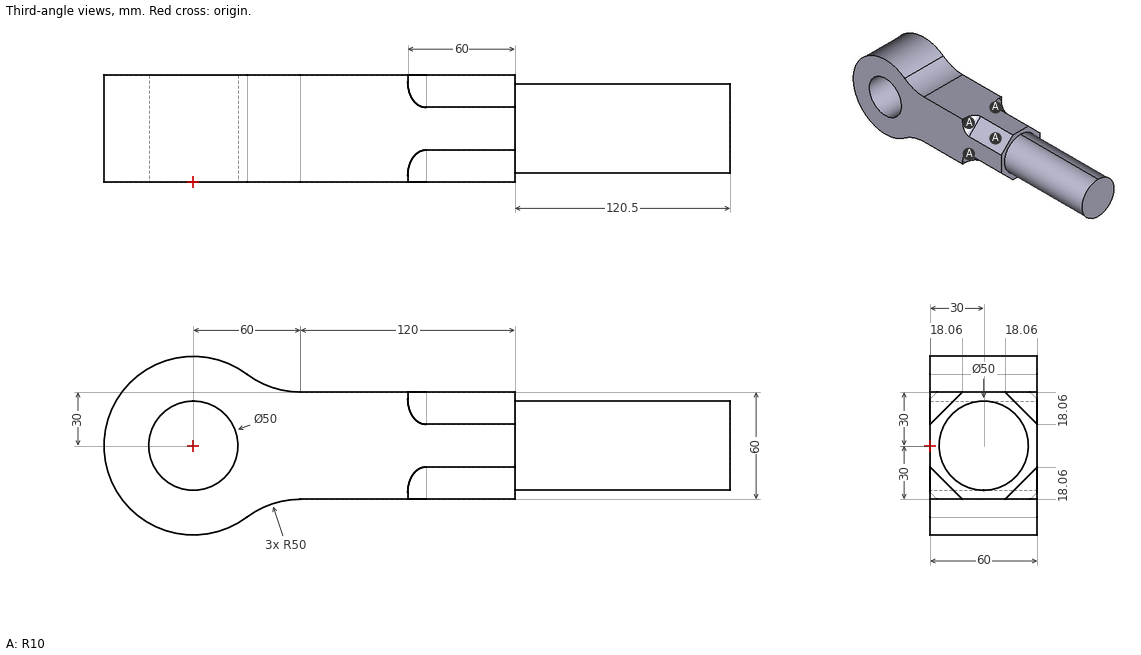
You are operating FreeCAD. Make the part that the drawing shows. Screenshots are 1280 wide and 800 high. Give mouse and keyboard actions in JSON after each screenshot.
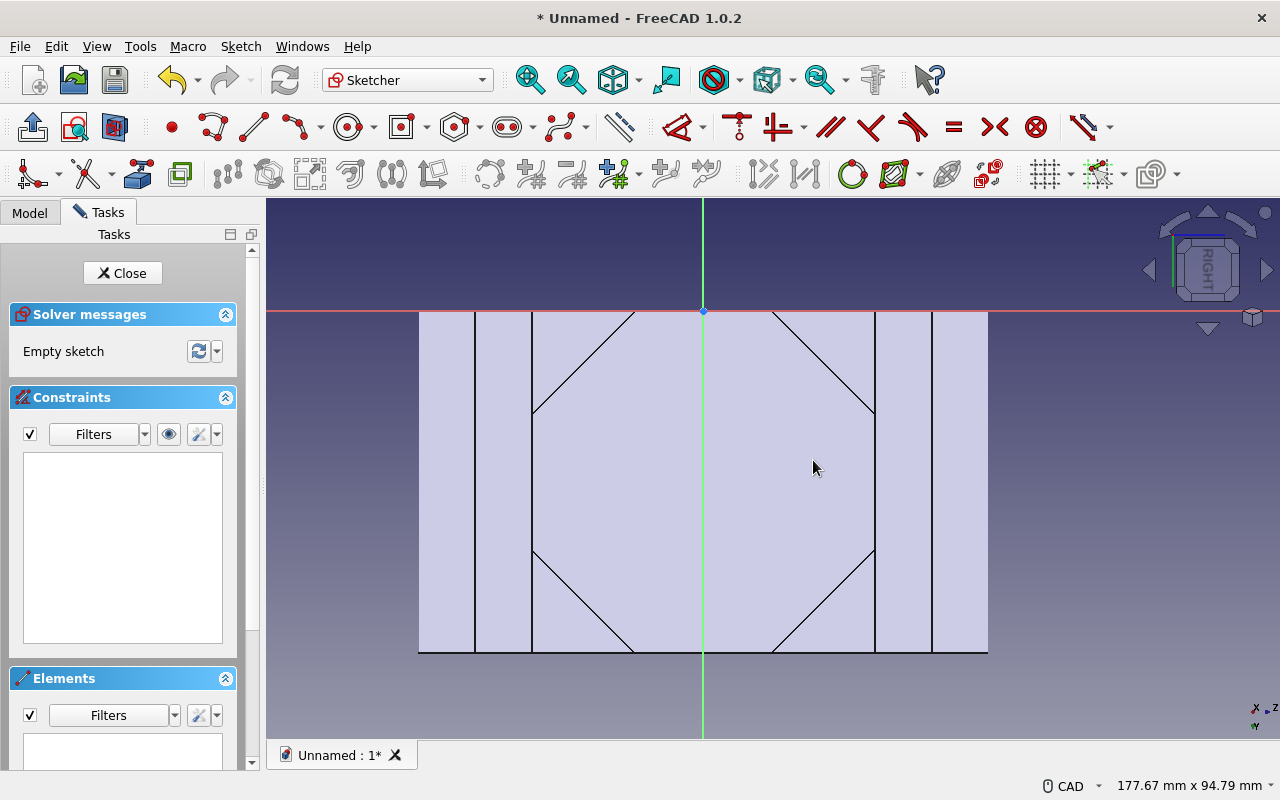
{"action": "key", "text": "g c"}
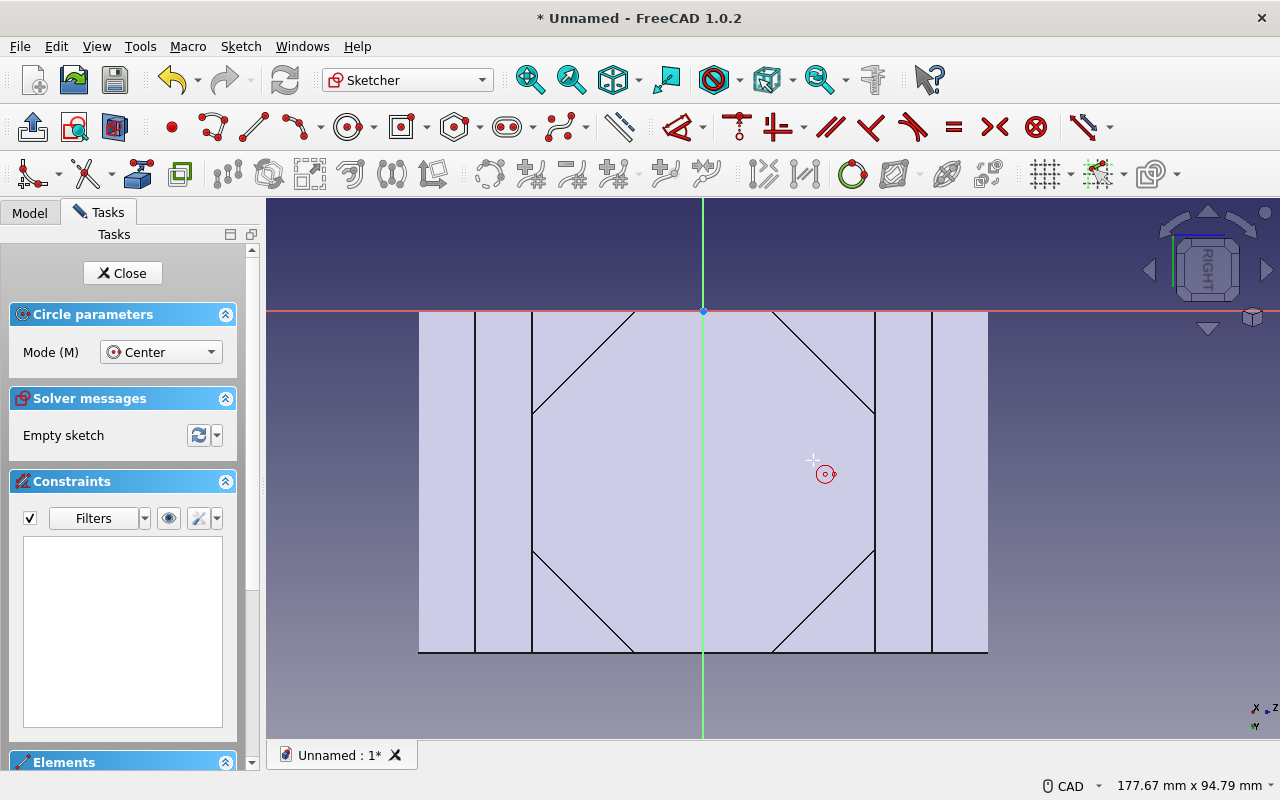
{"action": "left_click", "coordinate": [703, 482]}
{"action": "mouse_move", "coordinate": [804, 381]}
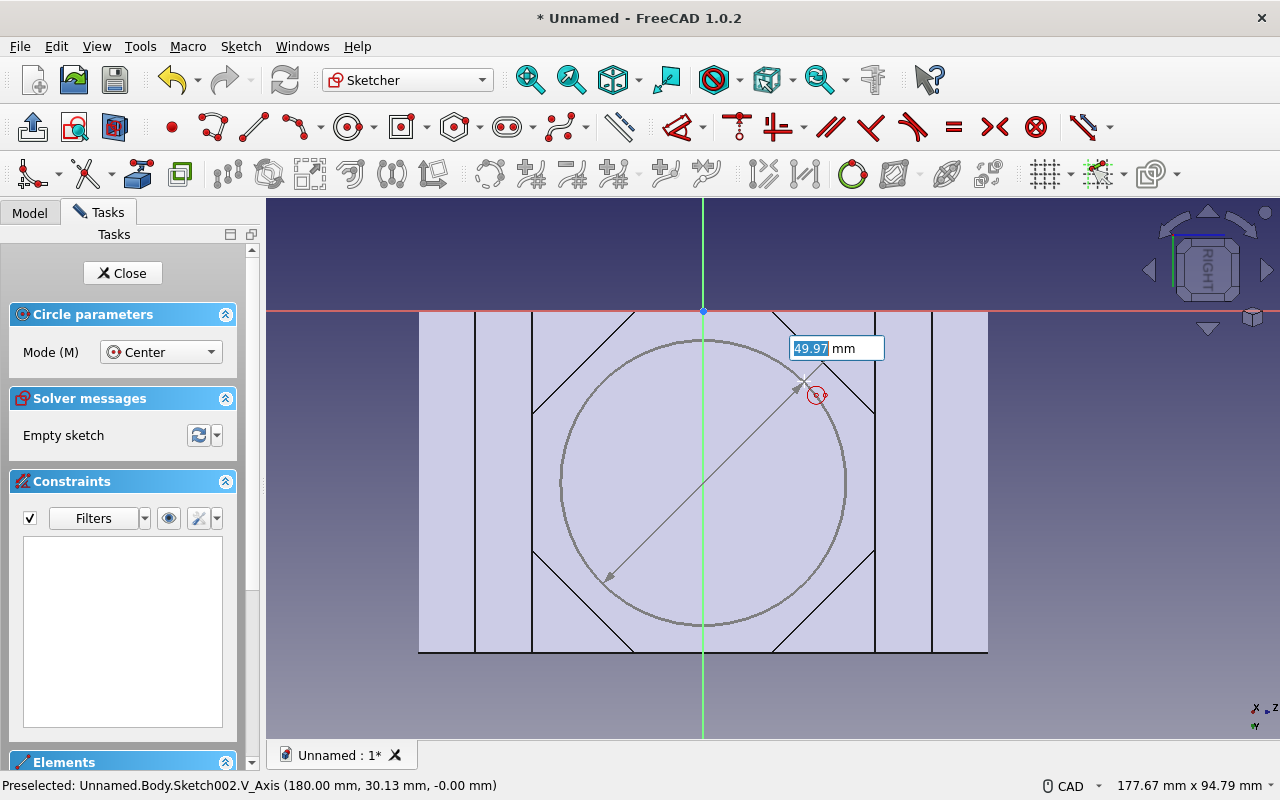
{"action": "type", "text": "50"}
{"action": "key", "text": "Return"}
{"action": "key", "text": "Escape"}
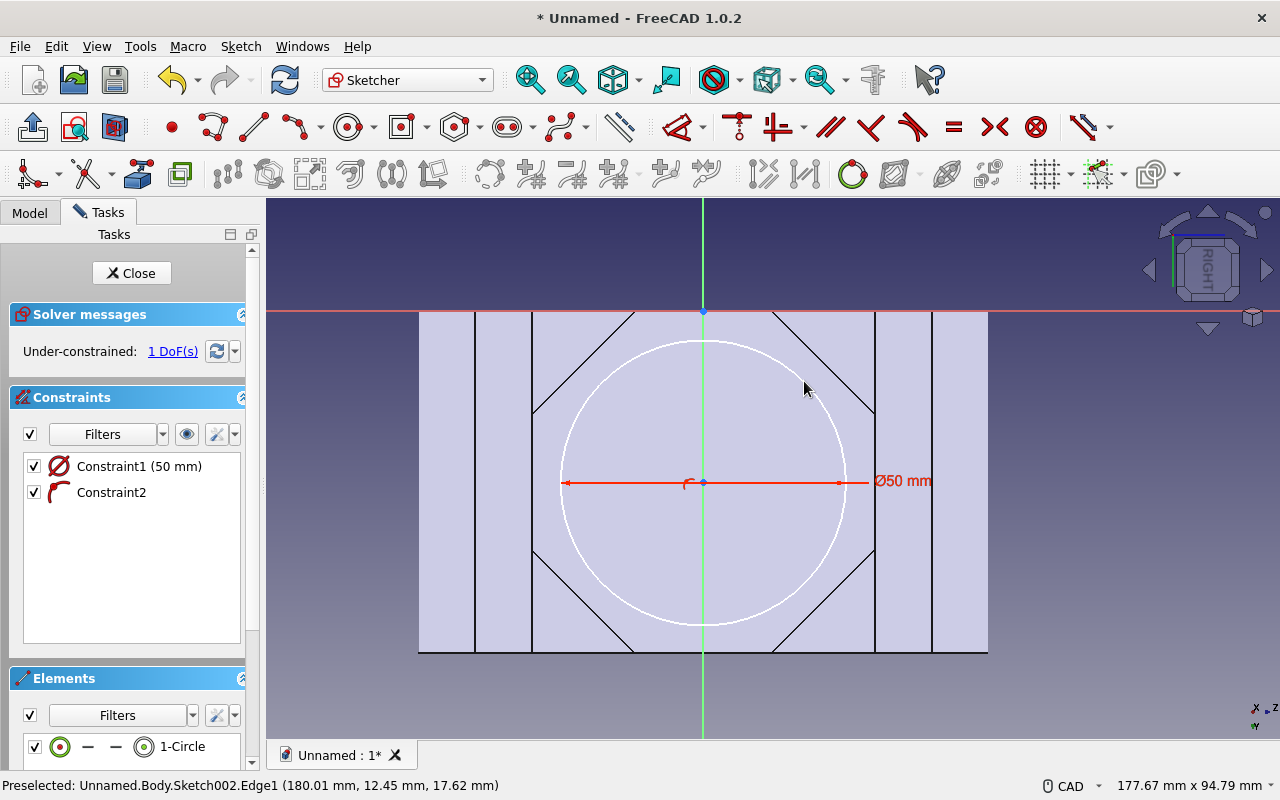
{"action": "key", "text": "d"}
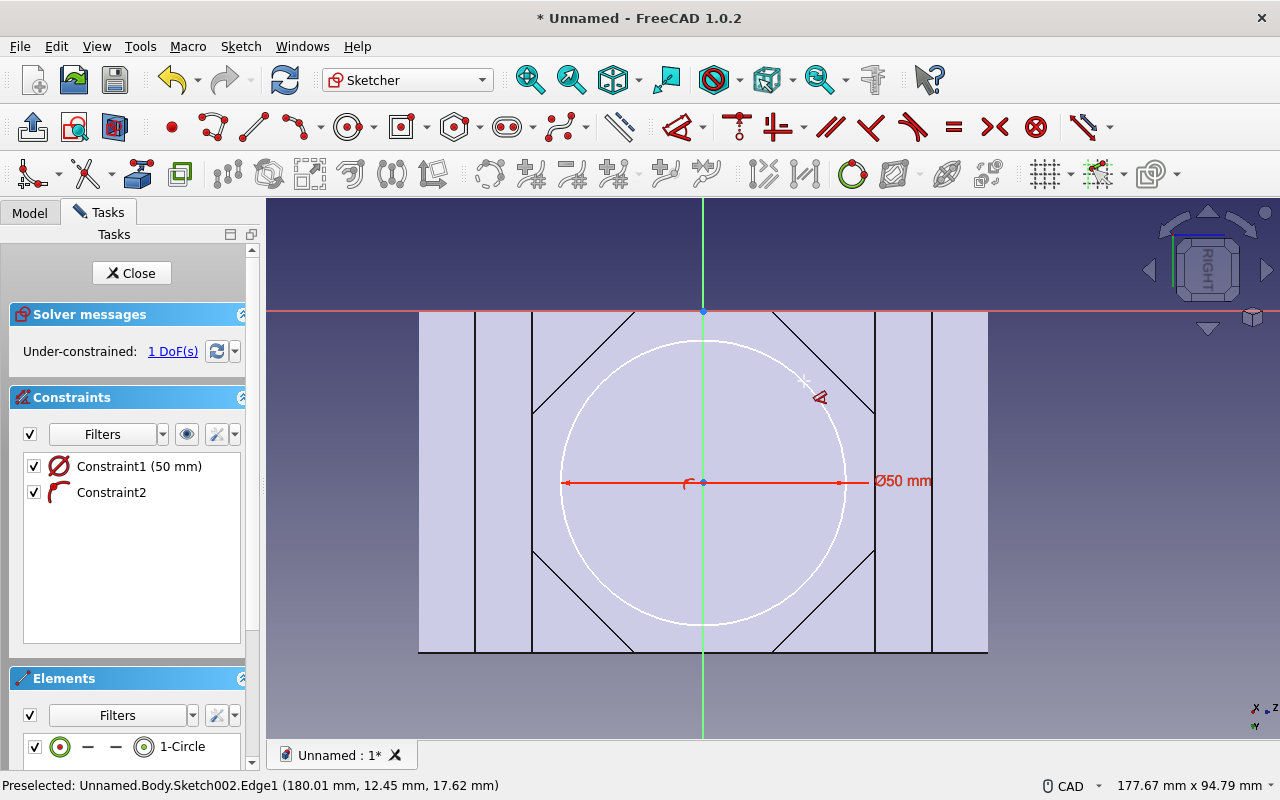
{"action": "left_click", "coordinate": [703, 483]}
{"action": "left_click", "coordinate": [737, 397]}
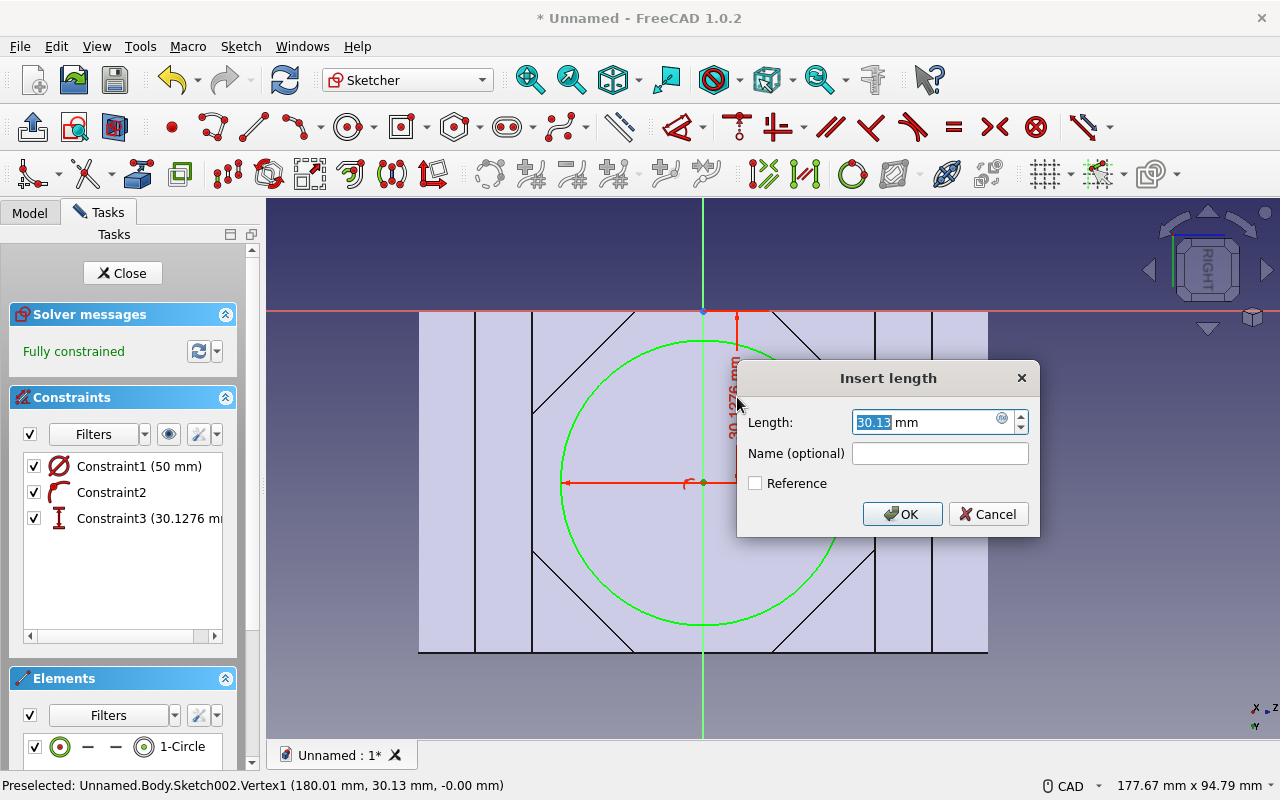
{"action": "type", "text": "30"}
{"action": "key", "text": "Return"}
{"action": "key", "text": "Escape"}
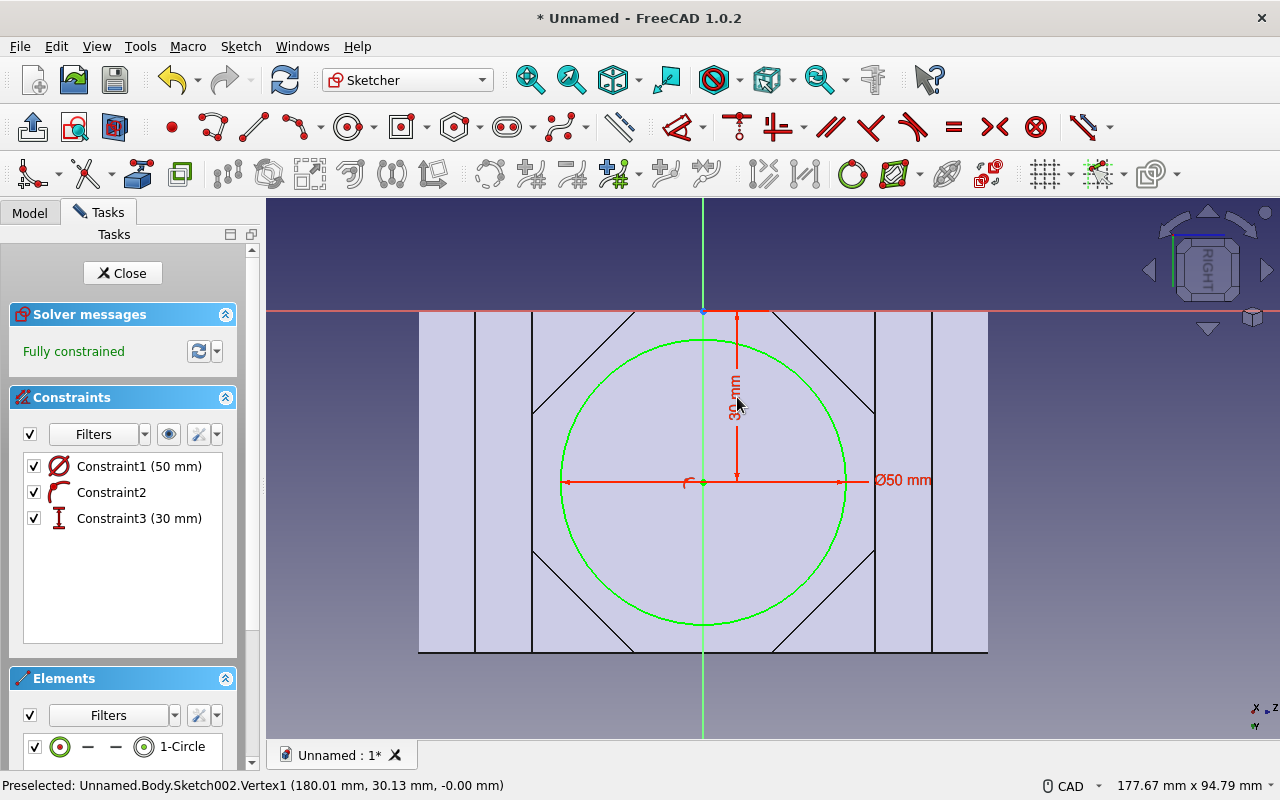
{"action": "left_click", "coordinate": [123, 273]}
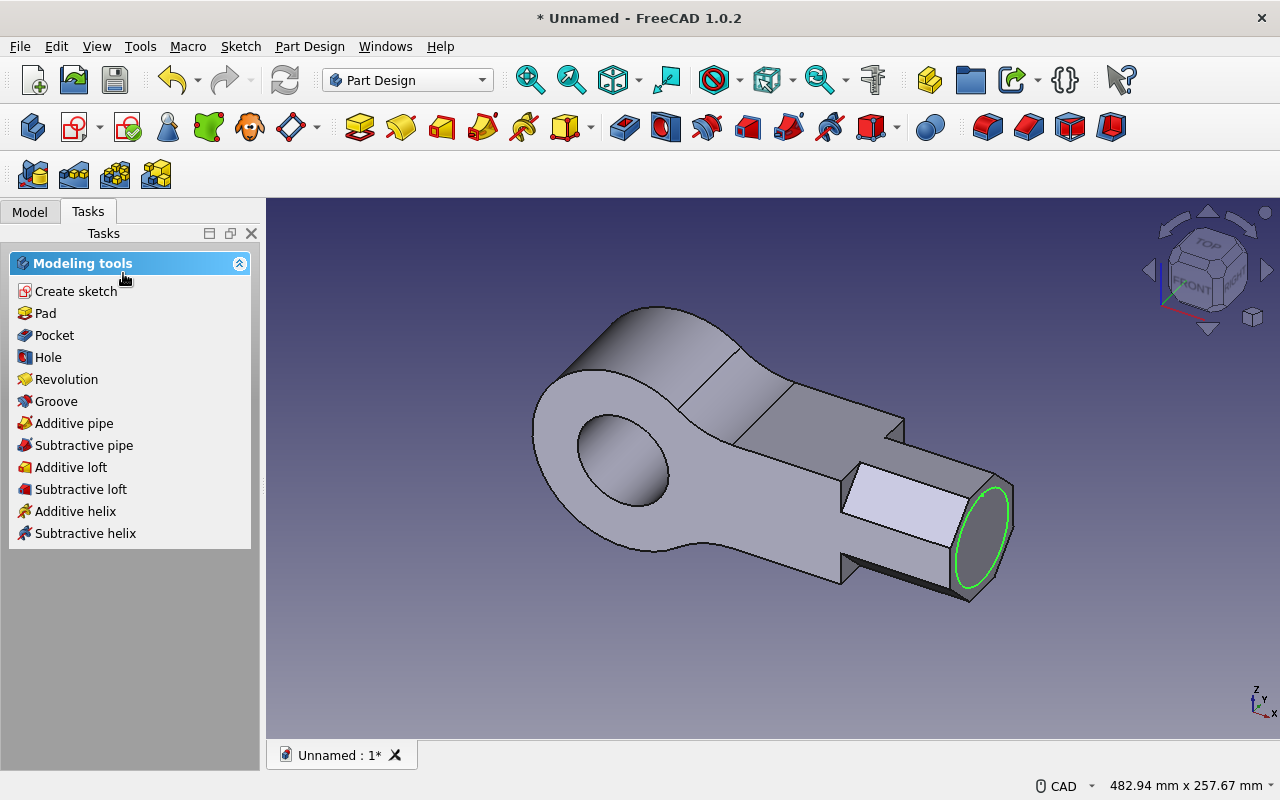
{"action": "left_click", "coordinate": [360, 128]}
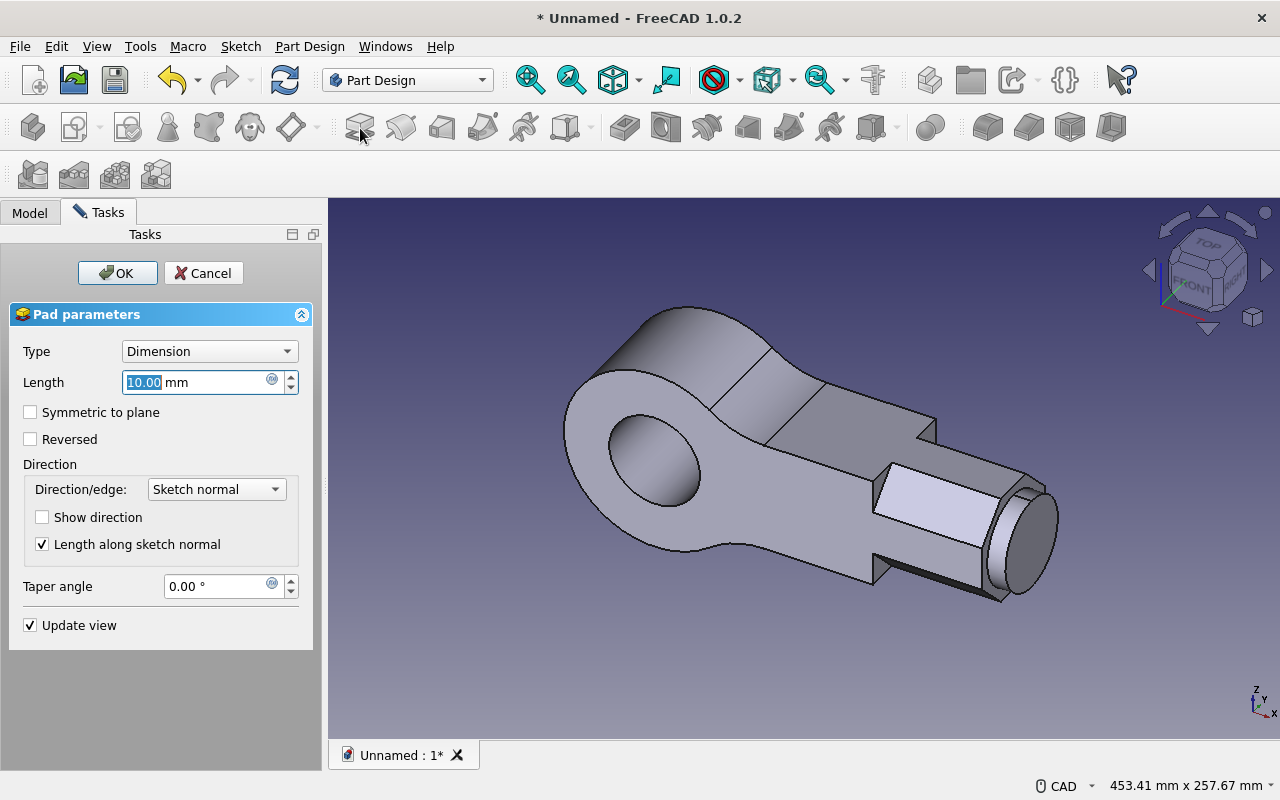
{"action": "type", "text": "120.5"}
{"action": "key", "text": "Tab"}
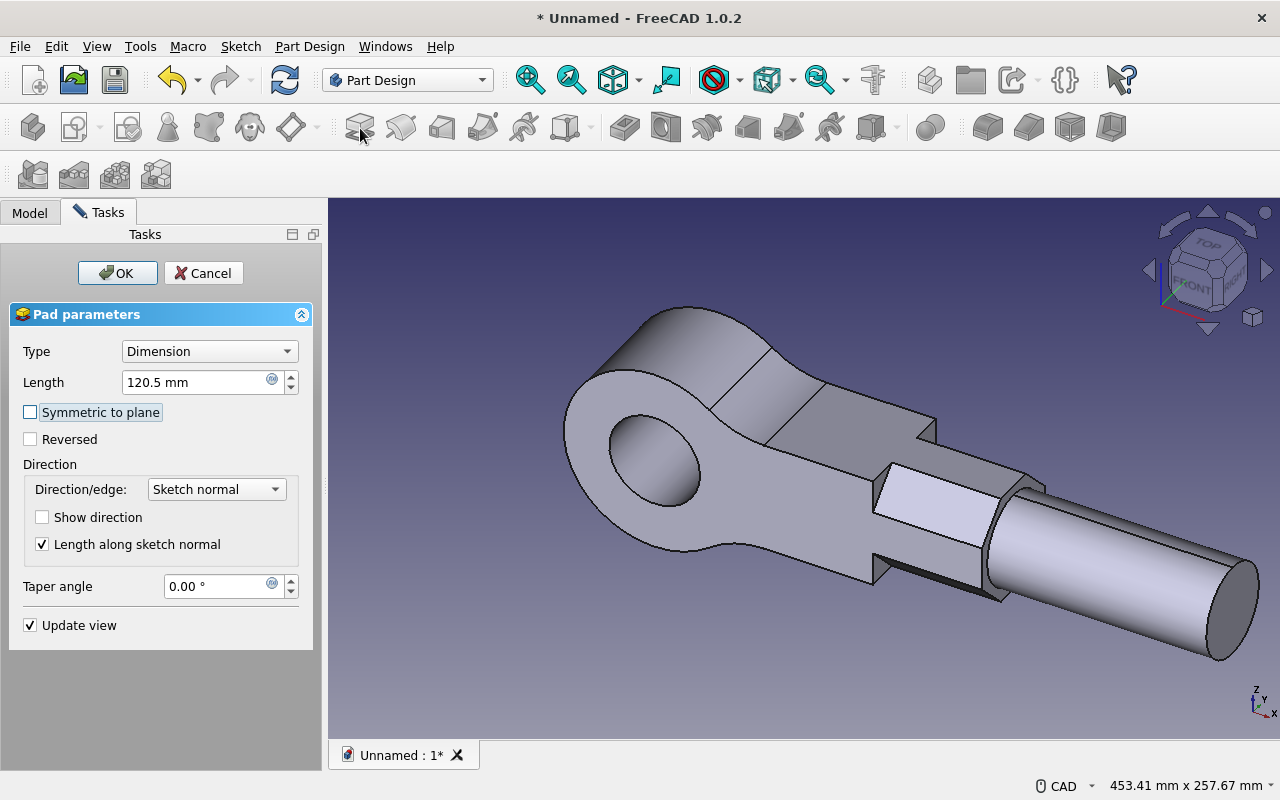
{"action": "left_click", "coordinate": [118, 273]}